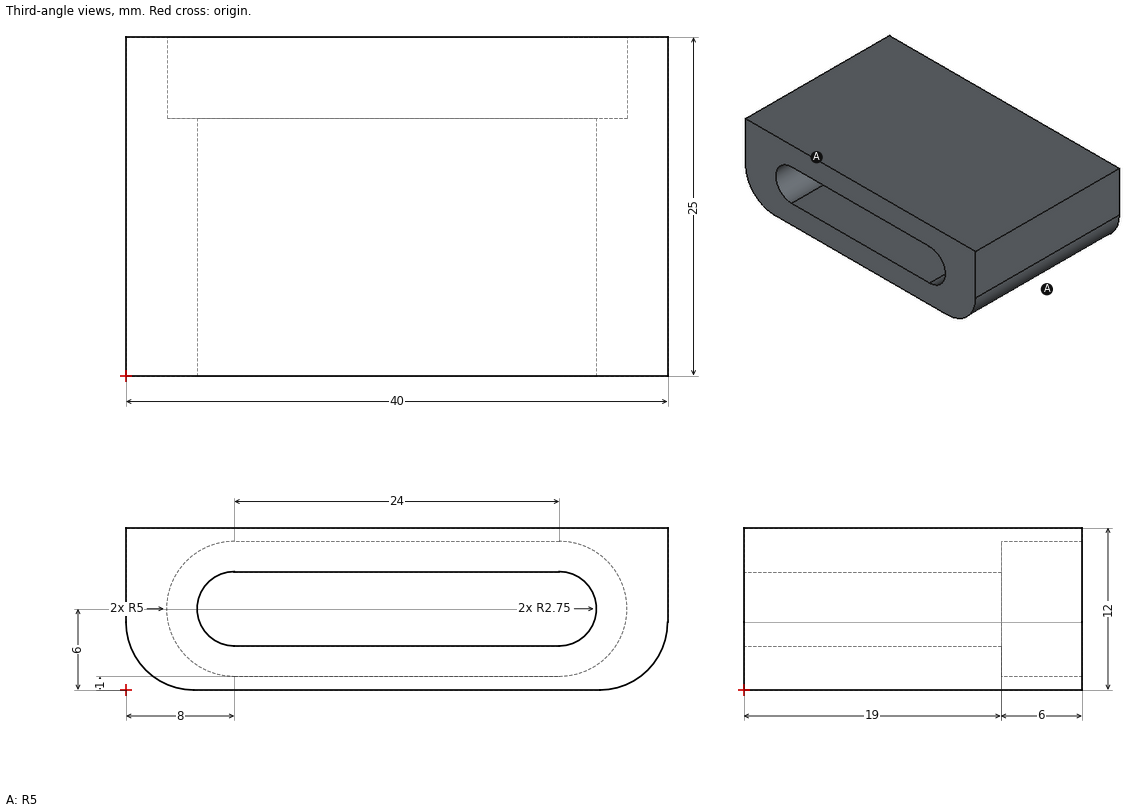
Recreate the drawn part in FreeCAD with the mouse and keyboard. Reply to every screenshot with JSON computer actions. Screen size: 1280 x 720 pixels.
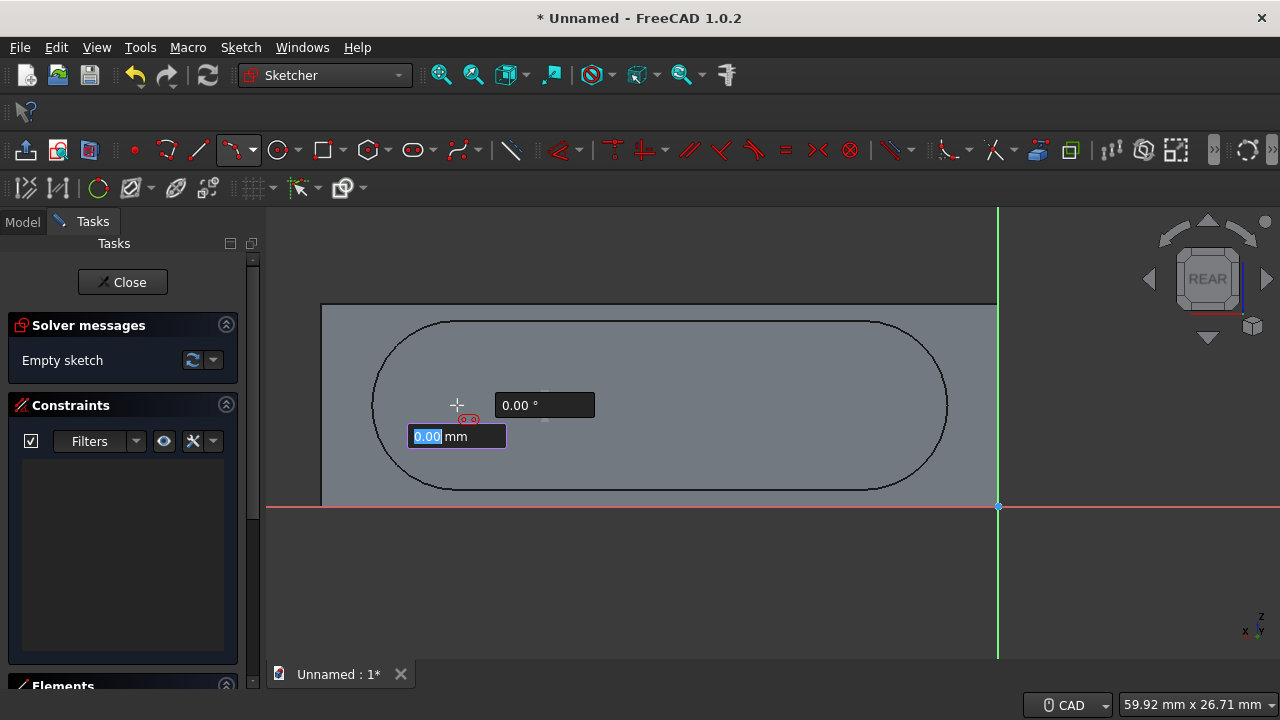
{"action": "left_click", "coordinate": [863, 405]}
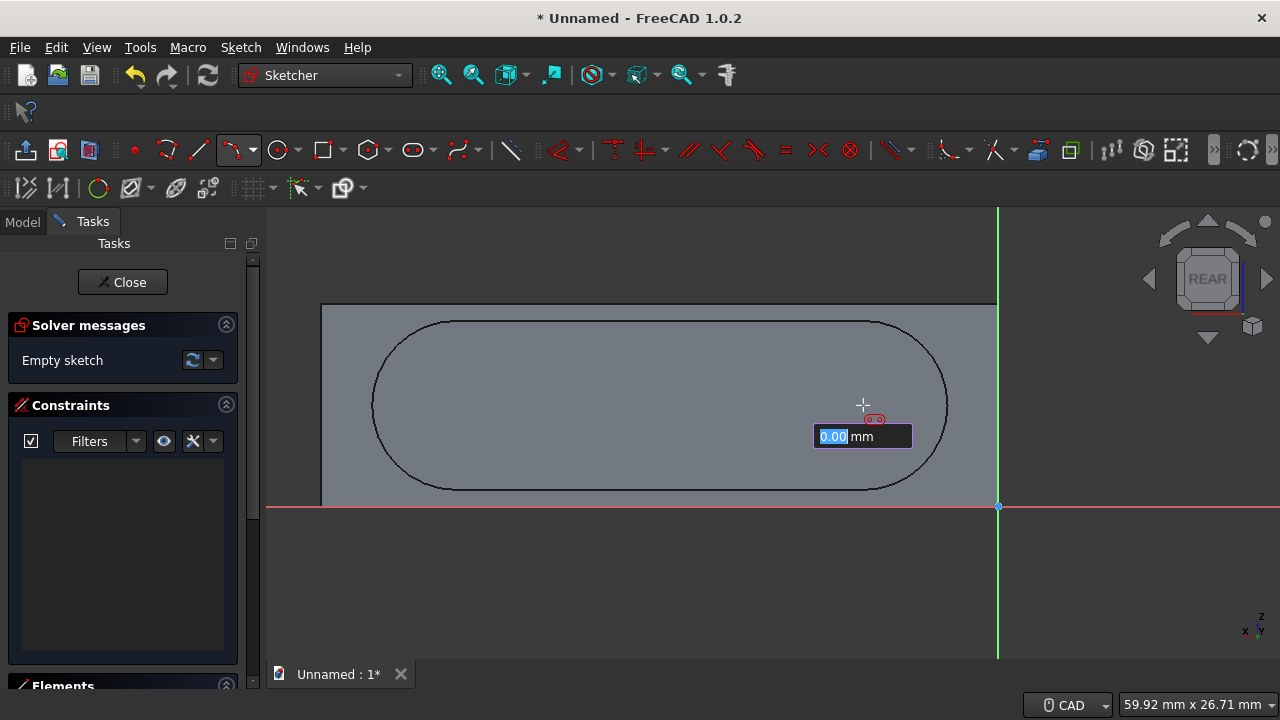
{"action": "left_click", "coordinate": [660, 359]}
{"action": "key", "text": "Escape"}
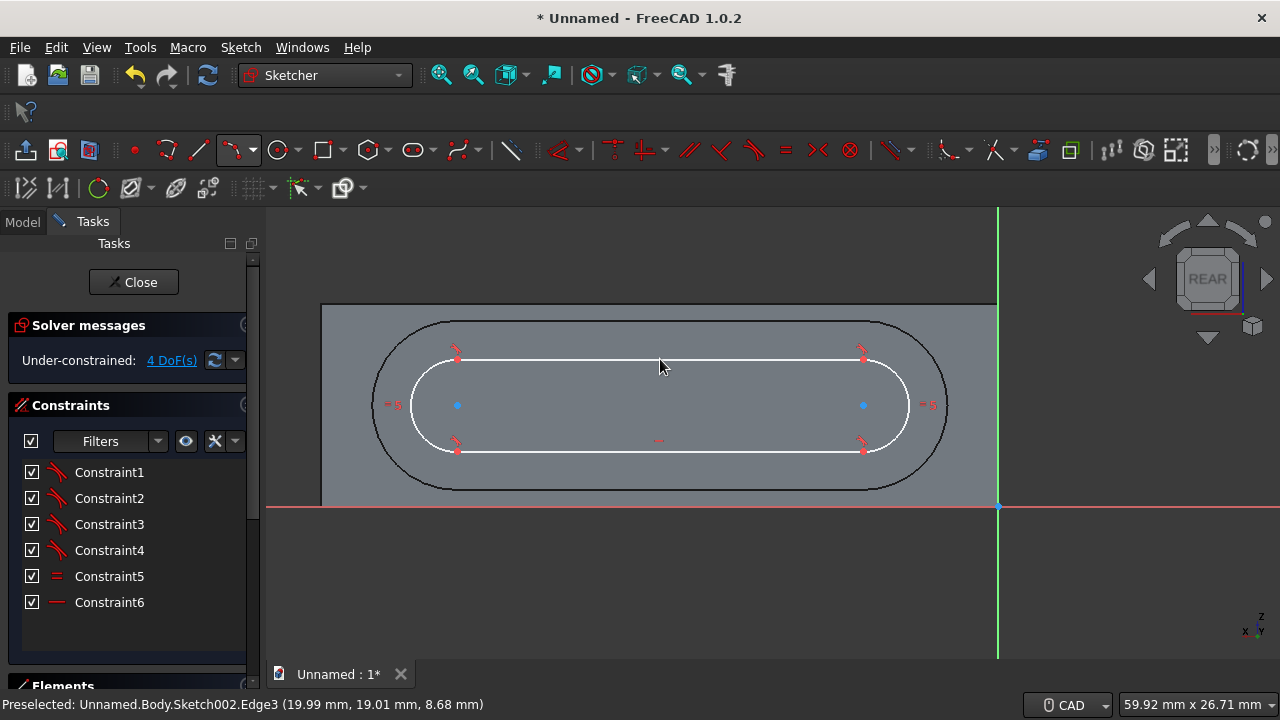
{"action": "key", "text": "d"}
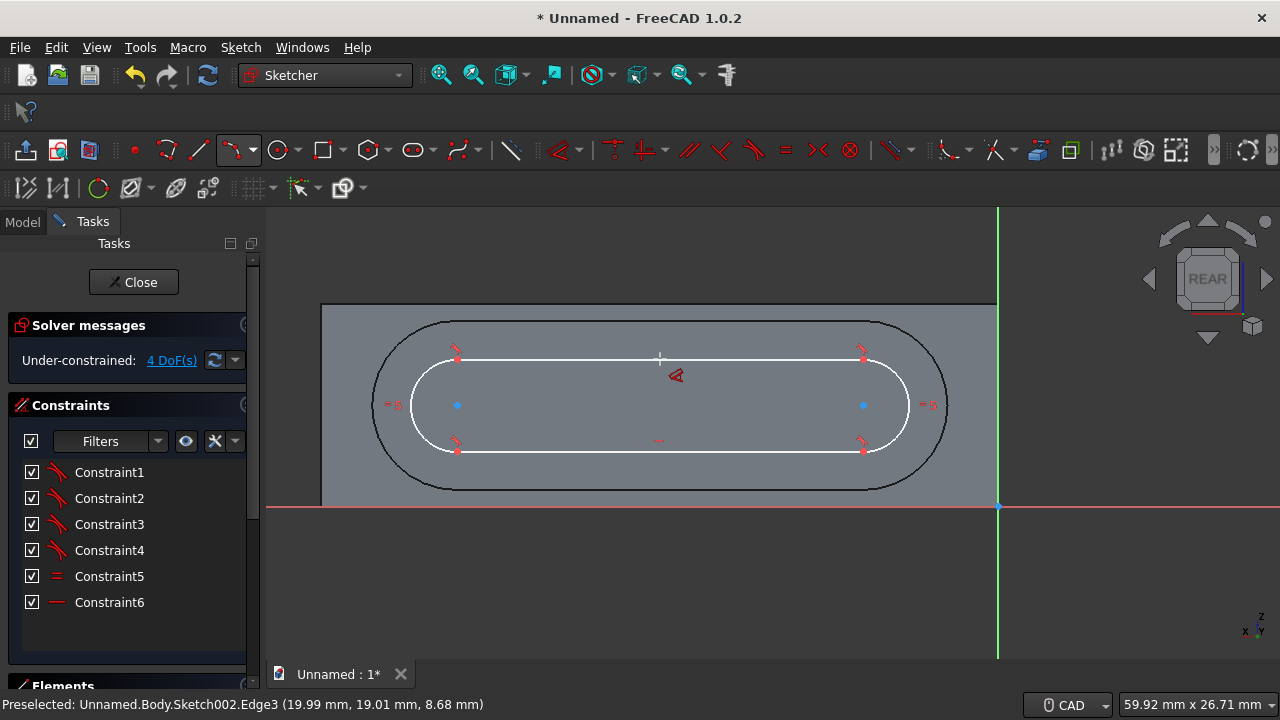
{"action": "left_click", "coordinate": [420, 379]}
{"action": "left_click", "coordinate": [394, 360]}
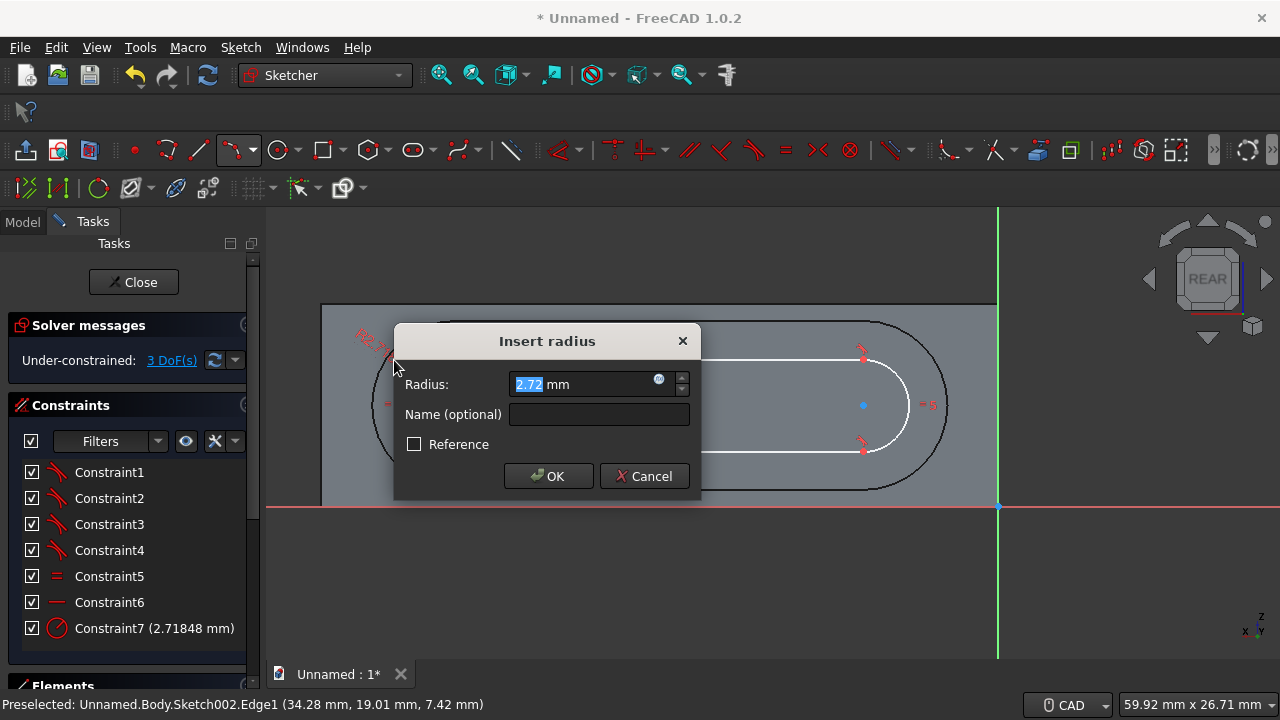
{"action": "type", "text": "2.75"}
{"action": "key", "text": "Return"}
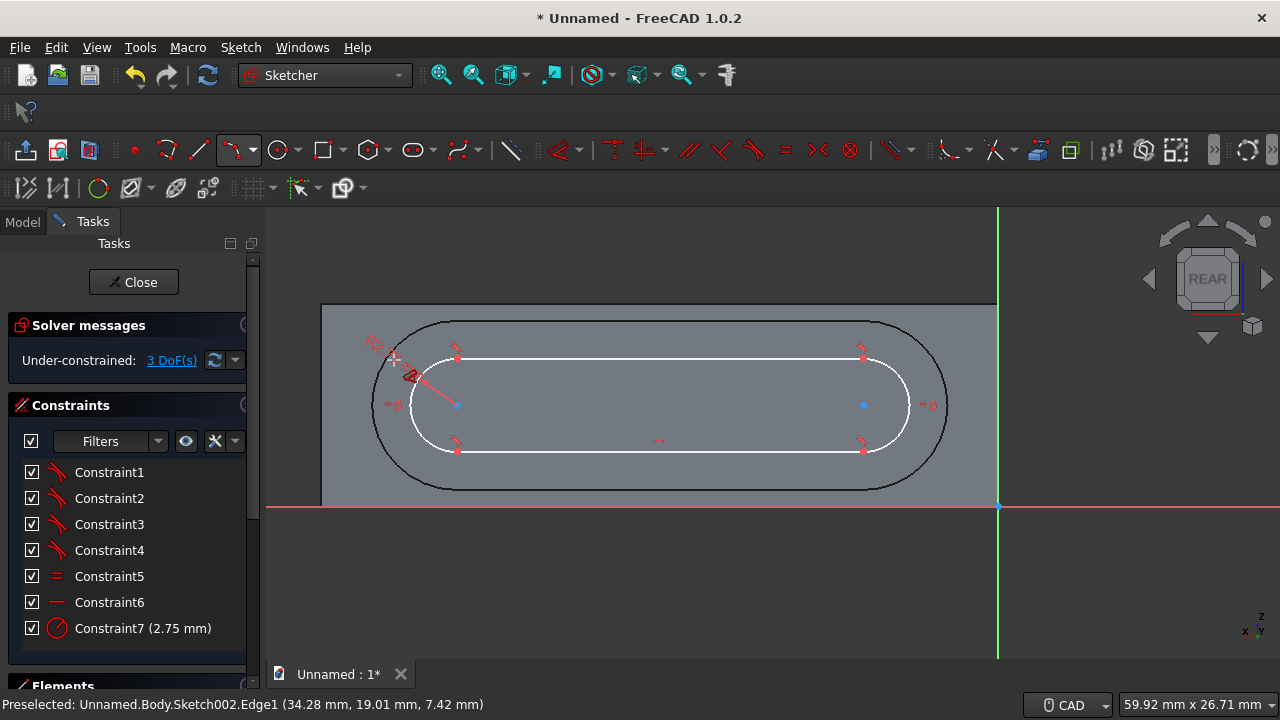
{"action": "left_click", "coordinate": [579, 359]}
{"action": "left_click", "coordinate": [660, 325]}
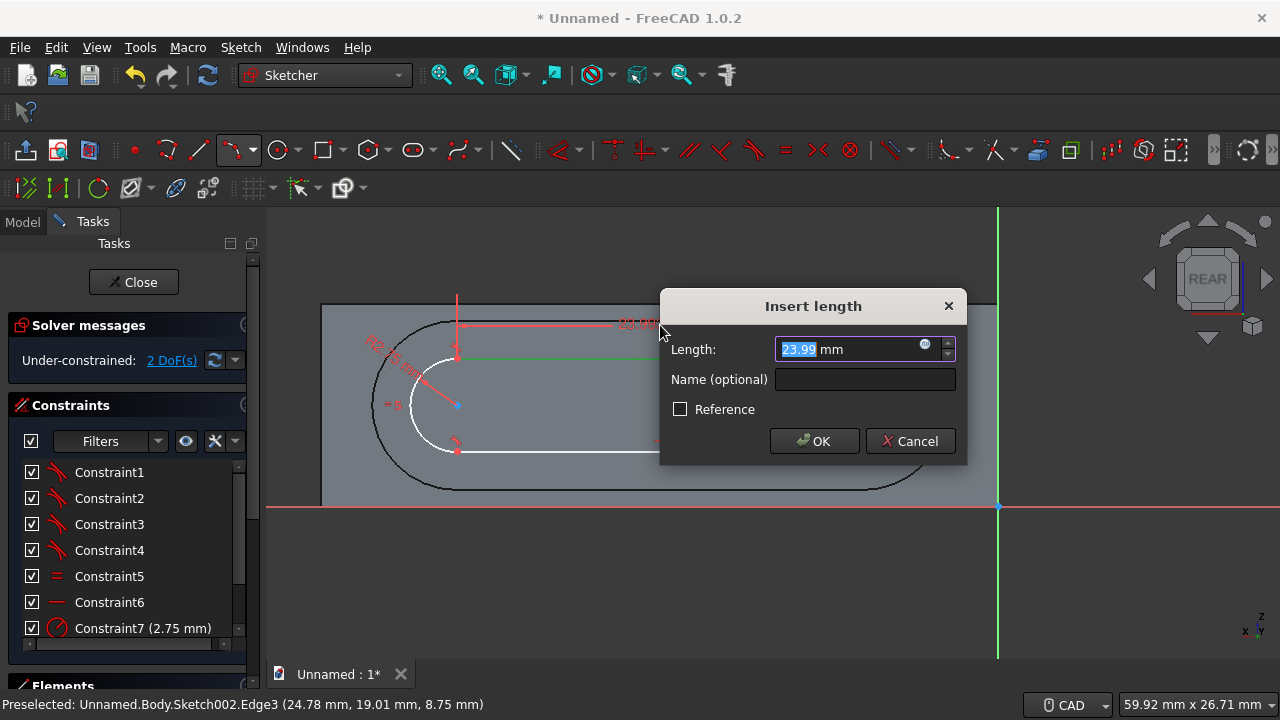
{"action": "type", "text": "24"}
{"action": "key", "text": "Return"}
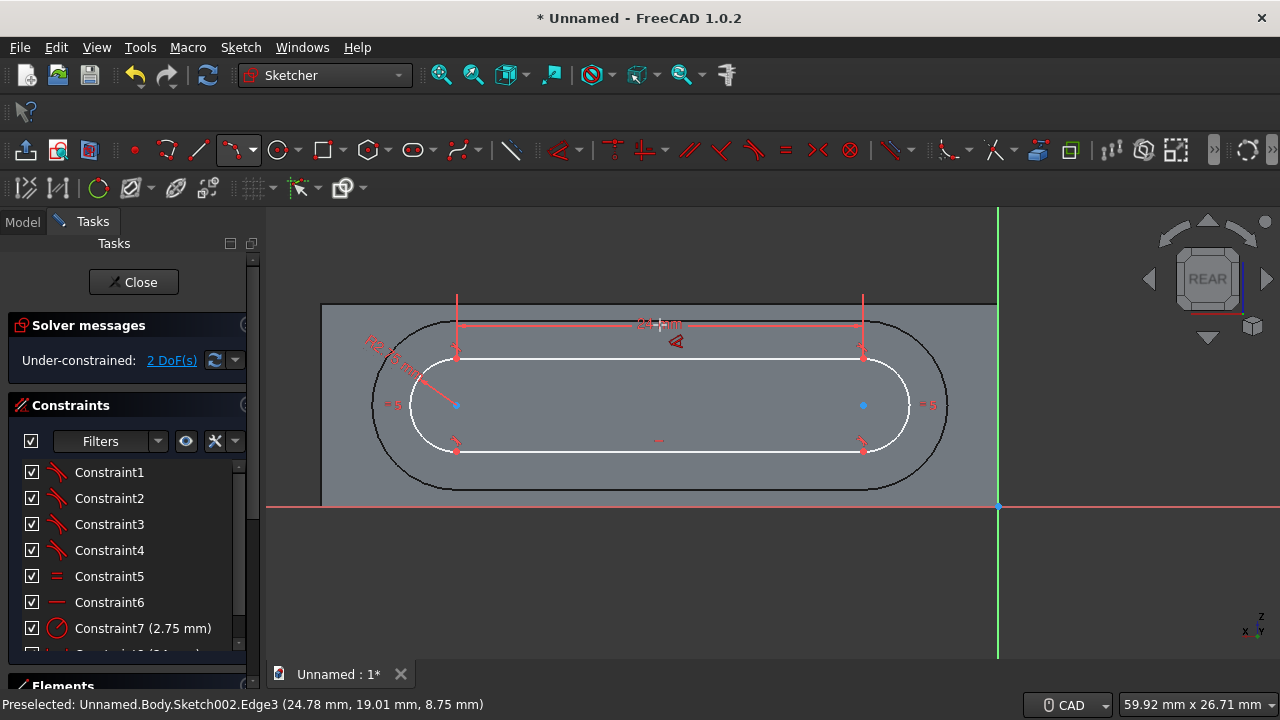
{"action": "left_click", "coordinate": [863, 452]}
{"action": "left_click", "coordinate": [931, 541]}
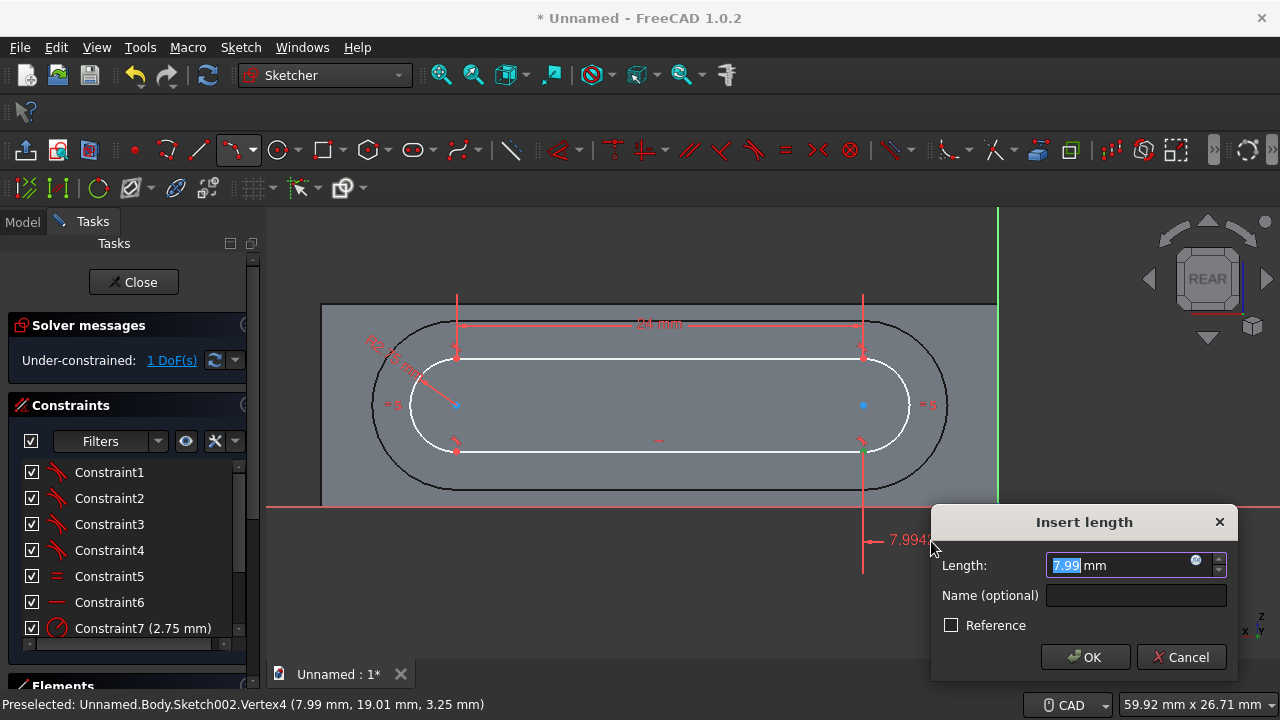
{"action": "type", "text": "8"}
{"action": "key", "text": "Return"}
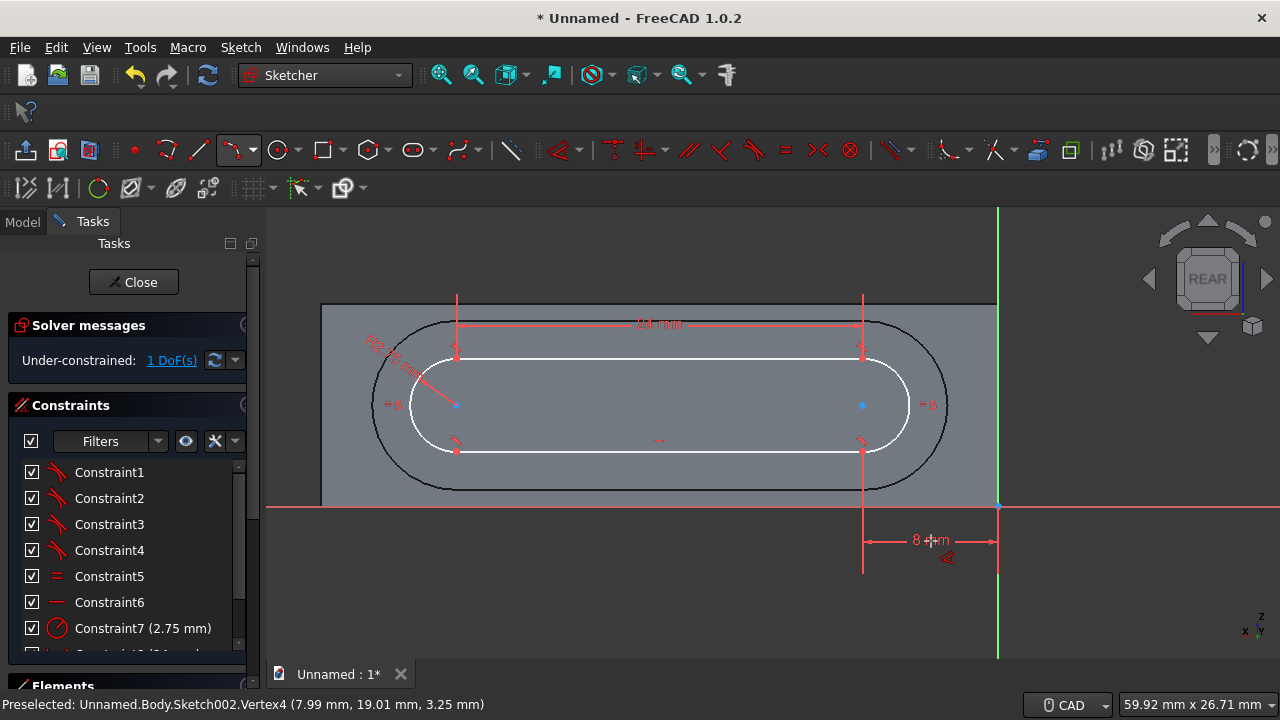
{"action": "left_click", "coordinate": [457, 405]}
{"action": "left_click", "coordinate": [1032, 456]}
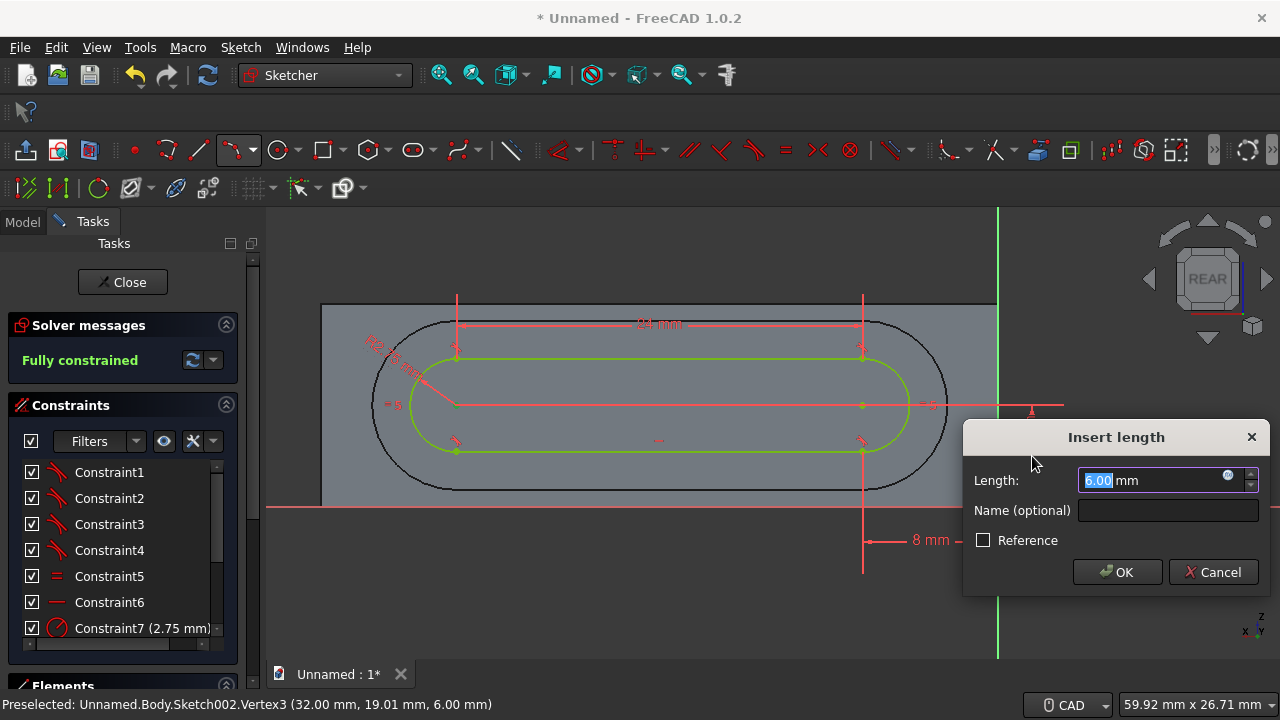
{"action": "type", "text": "6"}
{"action": "key", "text": "Return"}
{"action": "key", "text": "Escape"}